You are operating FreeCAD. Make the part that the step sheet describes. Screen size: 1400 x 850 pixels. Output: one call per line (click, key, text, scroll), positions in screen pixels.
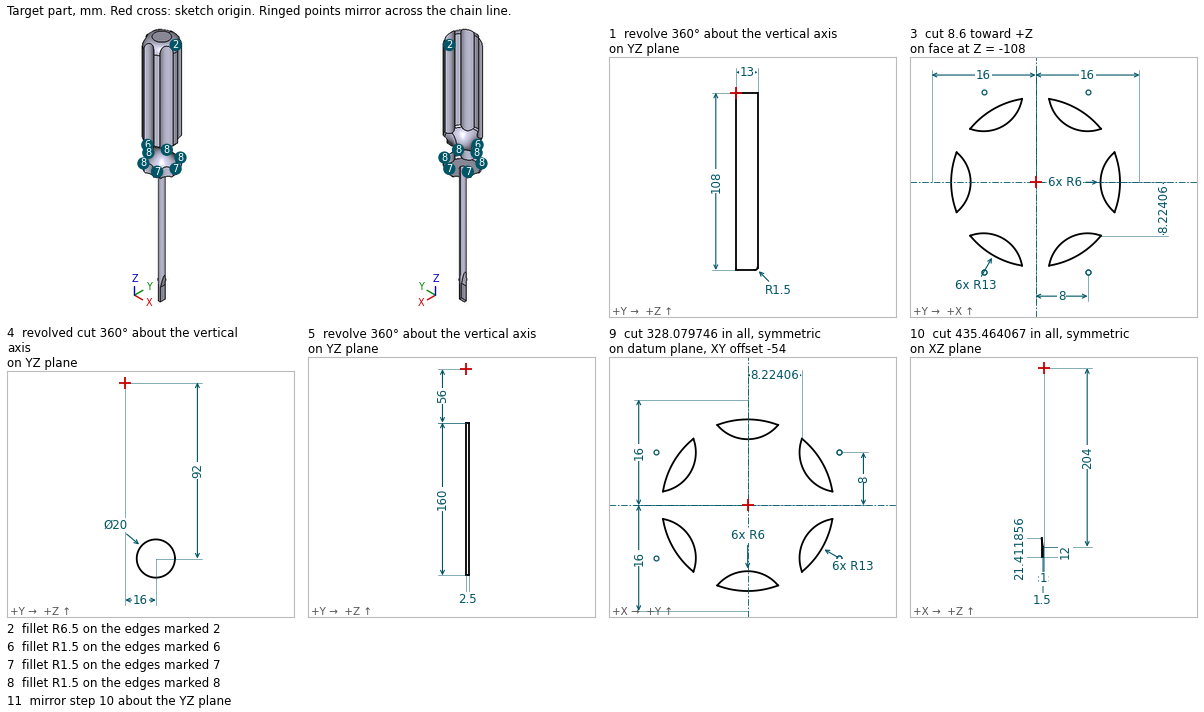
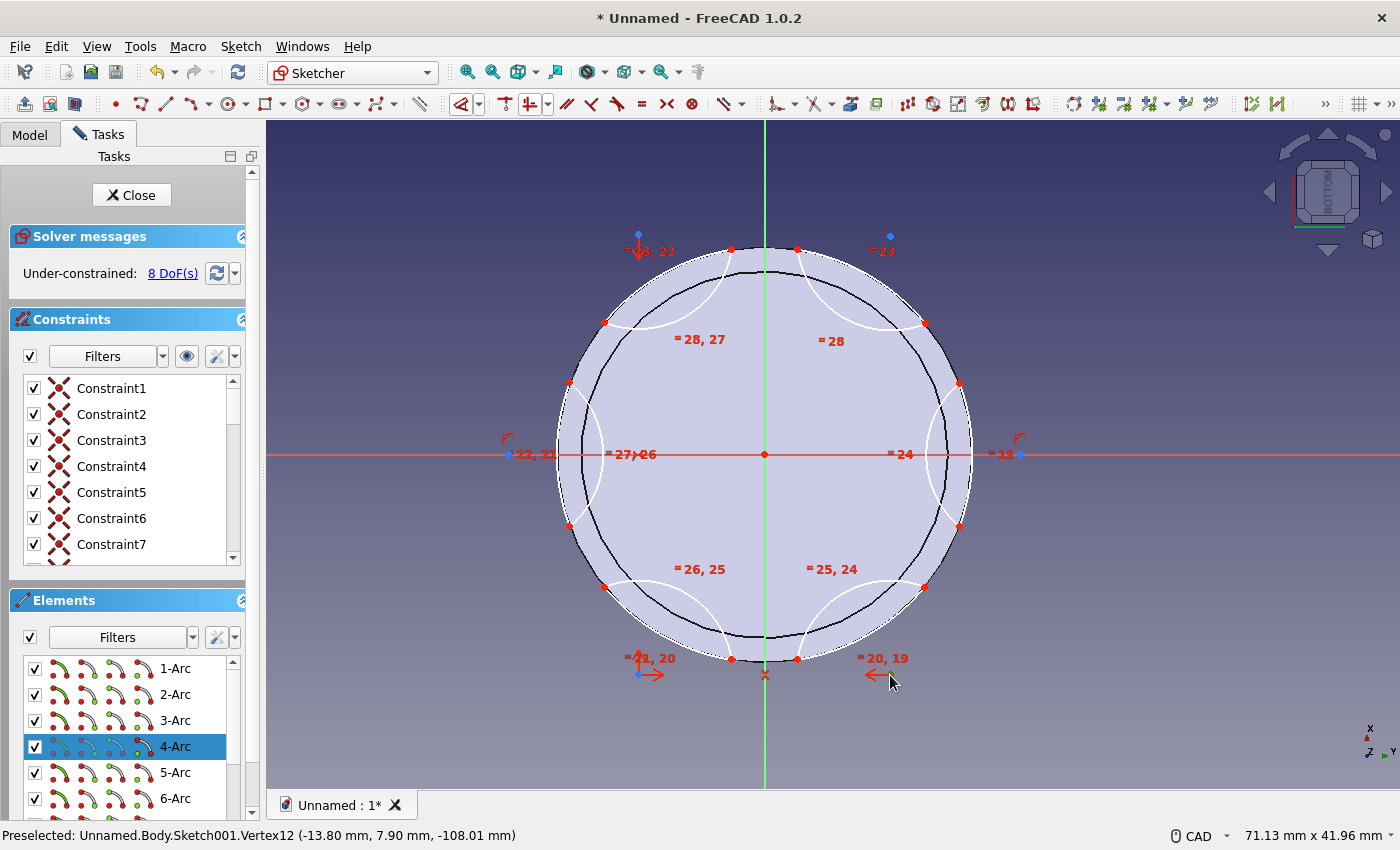
click(891, 236)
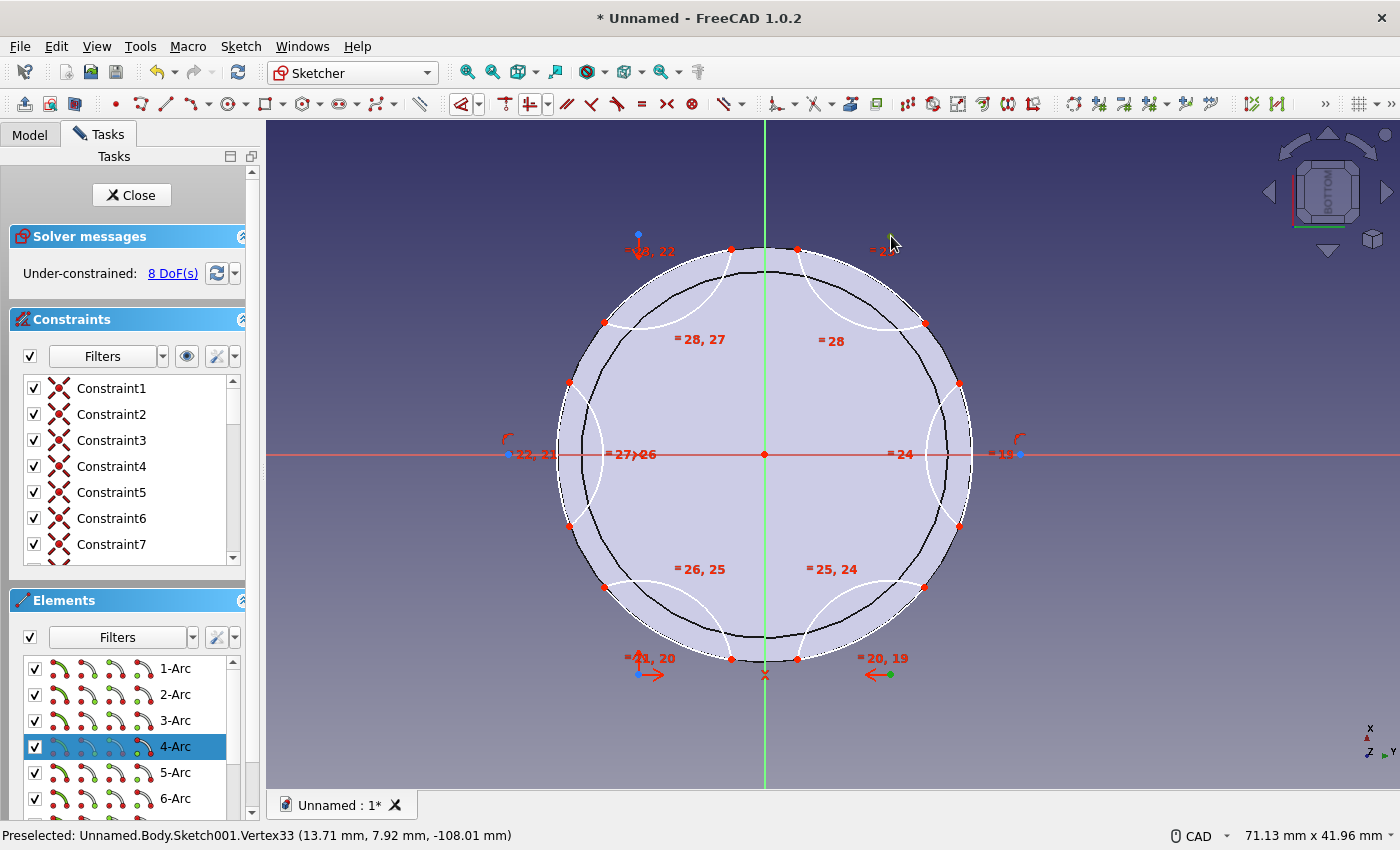
click(361, 455)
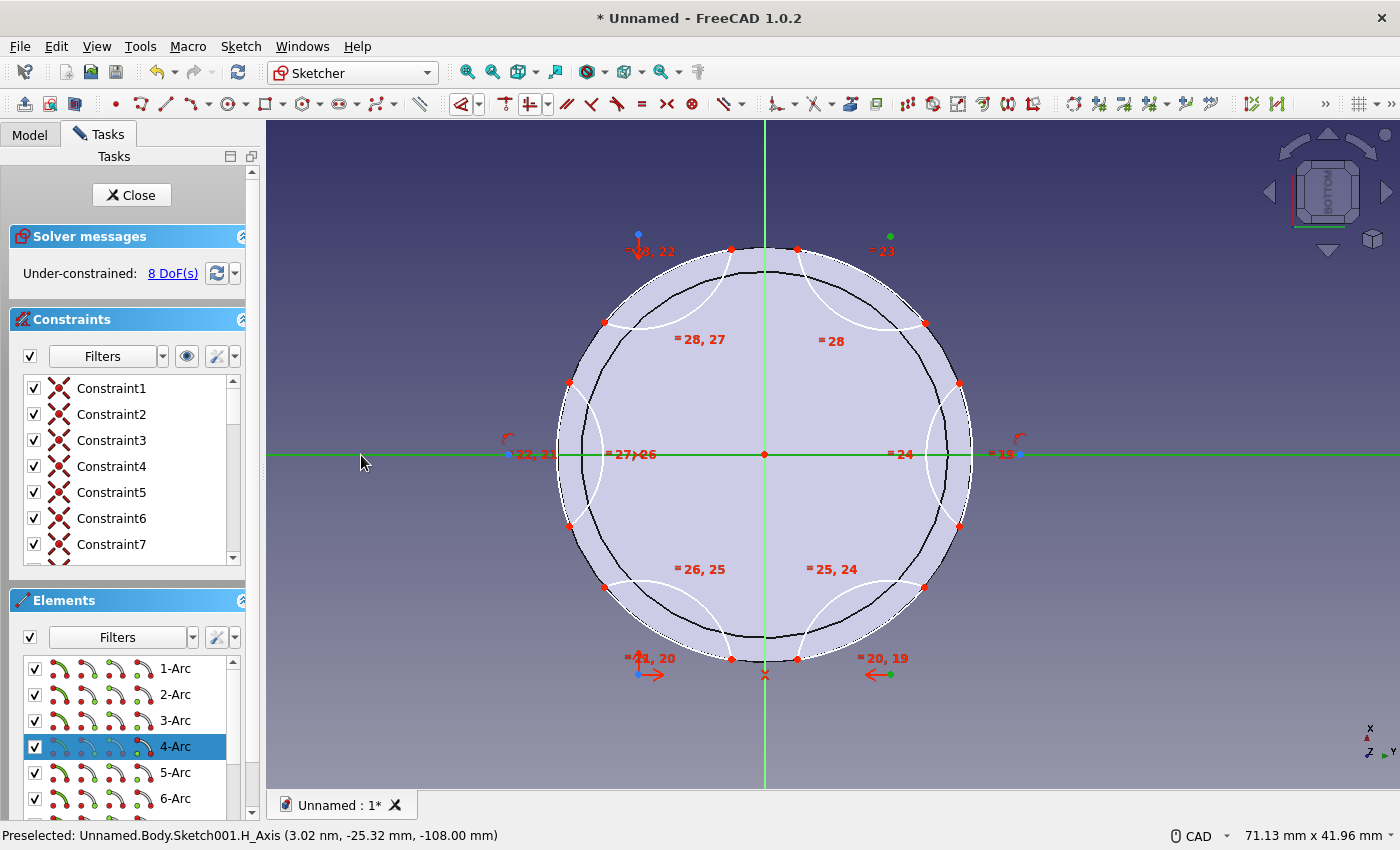
key(s)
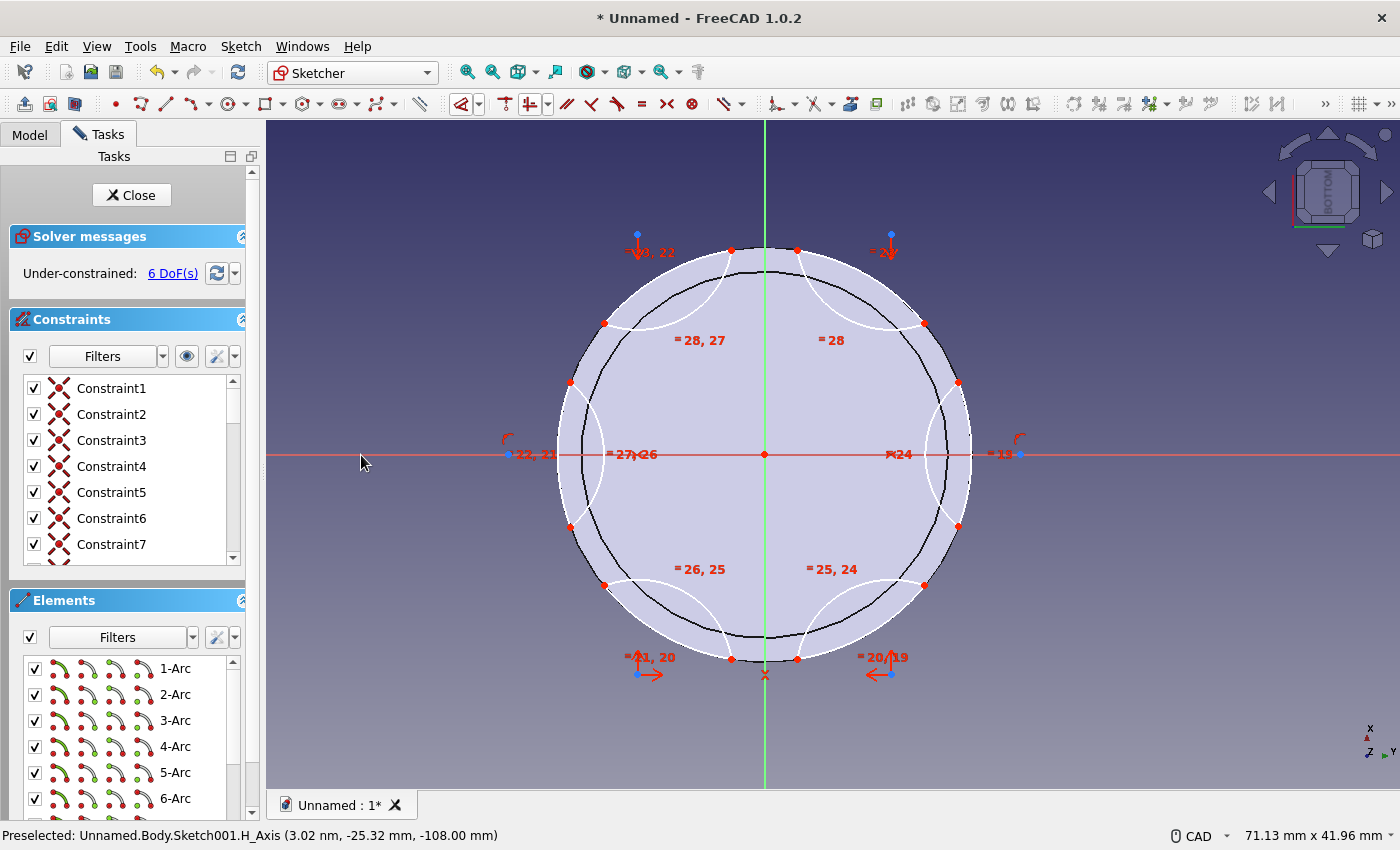
key(d)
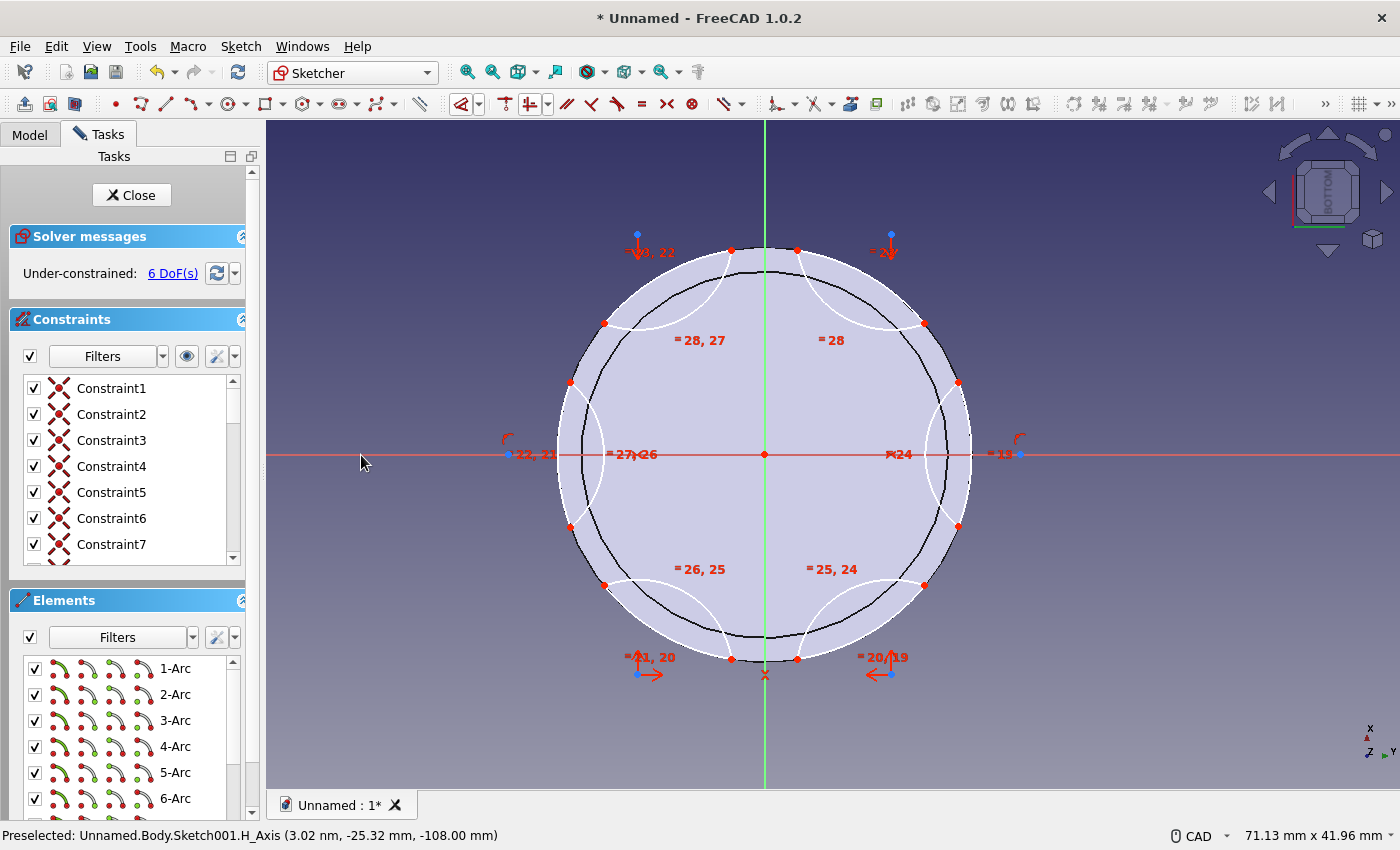
click(931, 423)
click(901, 412)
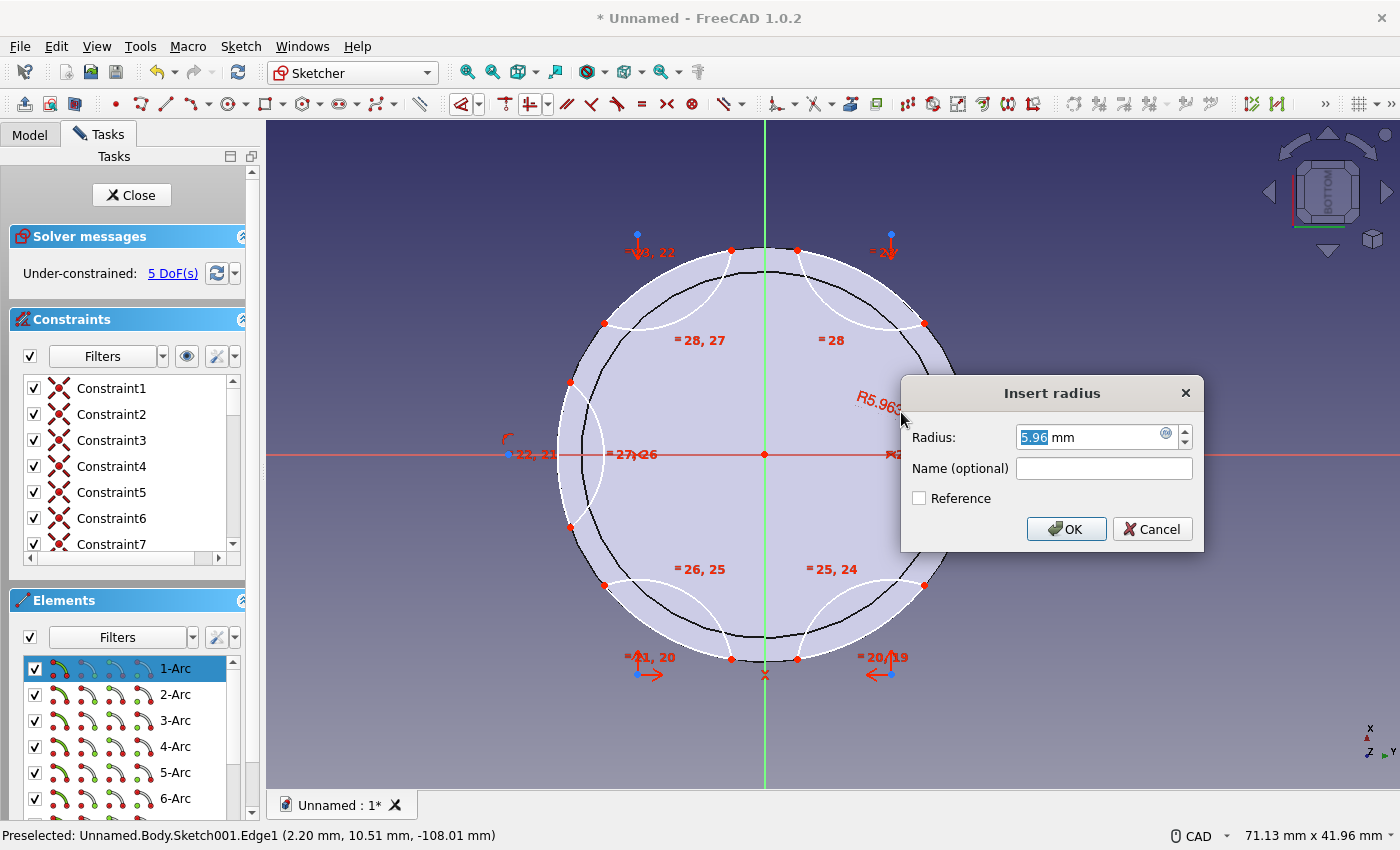
text(6)
key(Return)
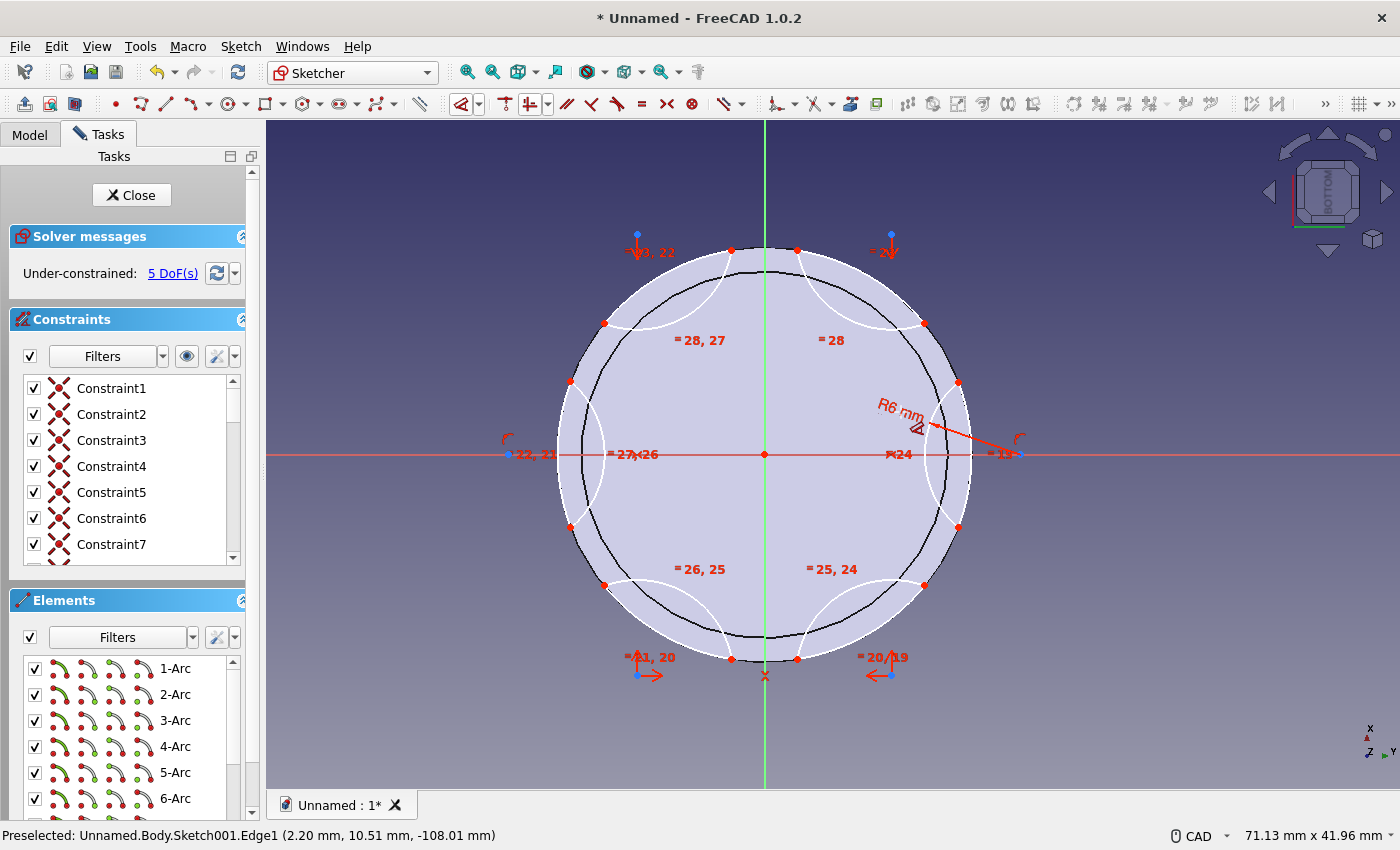
click(969, 484)
click(1001, 489)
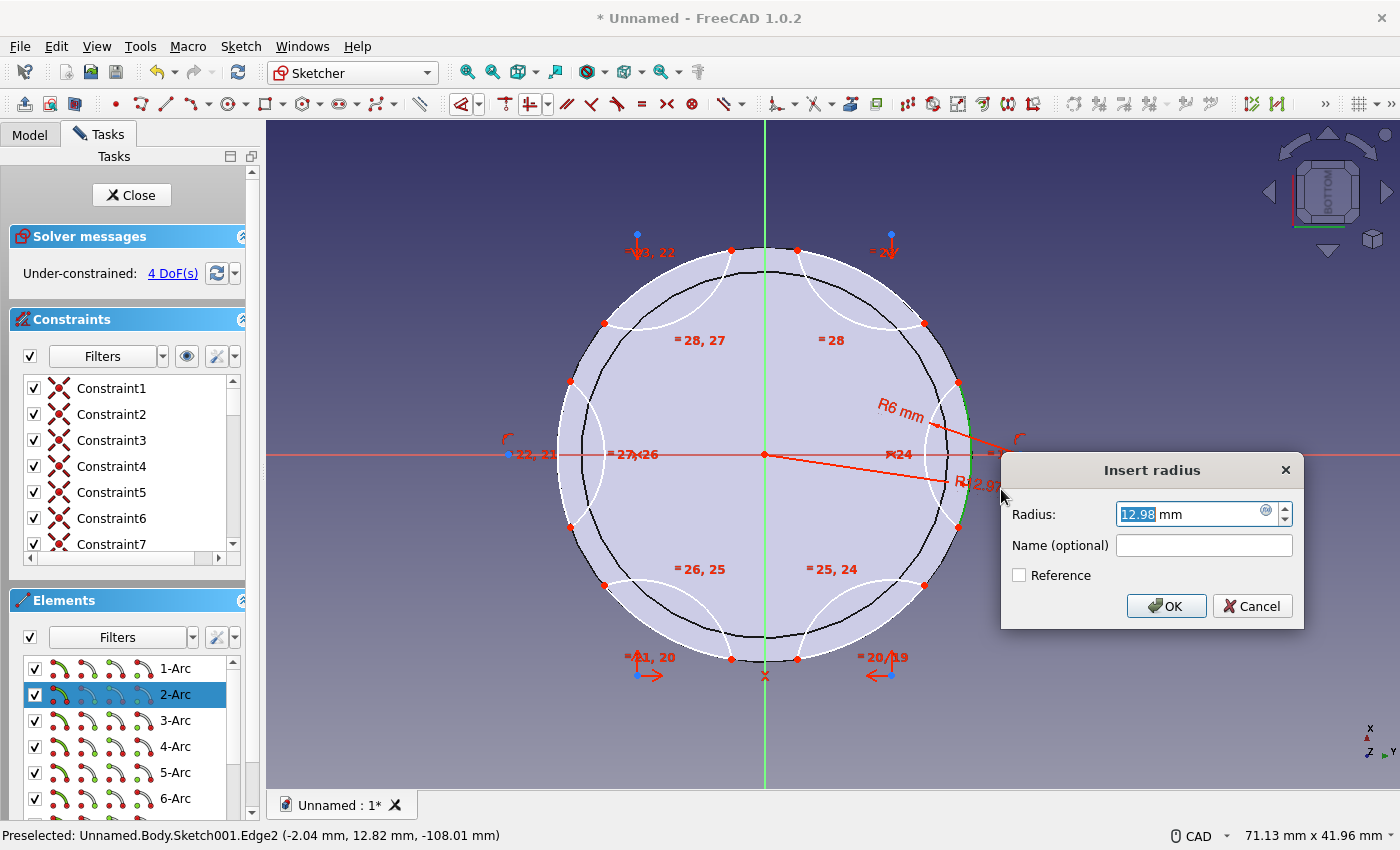
text(13)
key(Return)